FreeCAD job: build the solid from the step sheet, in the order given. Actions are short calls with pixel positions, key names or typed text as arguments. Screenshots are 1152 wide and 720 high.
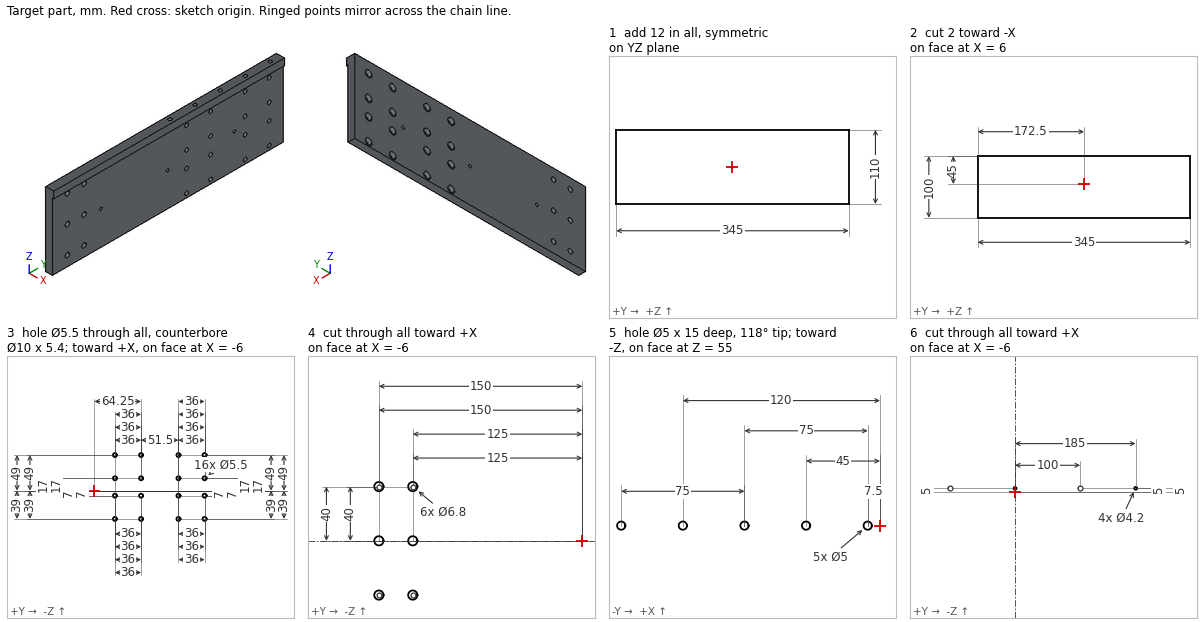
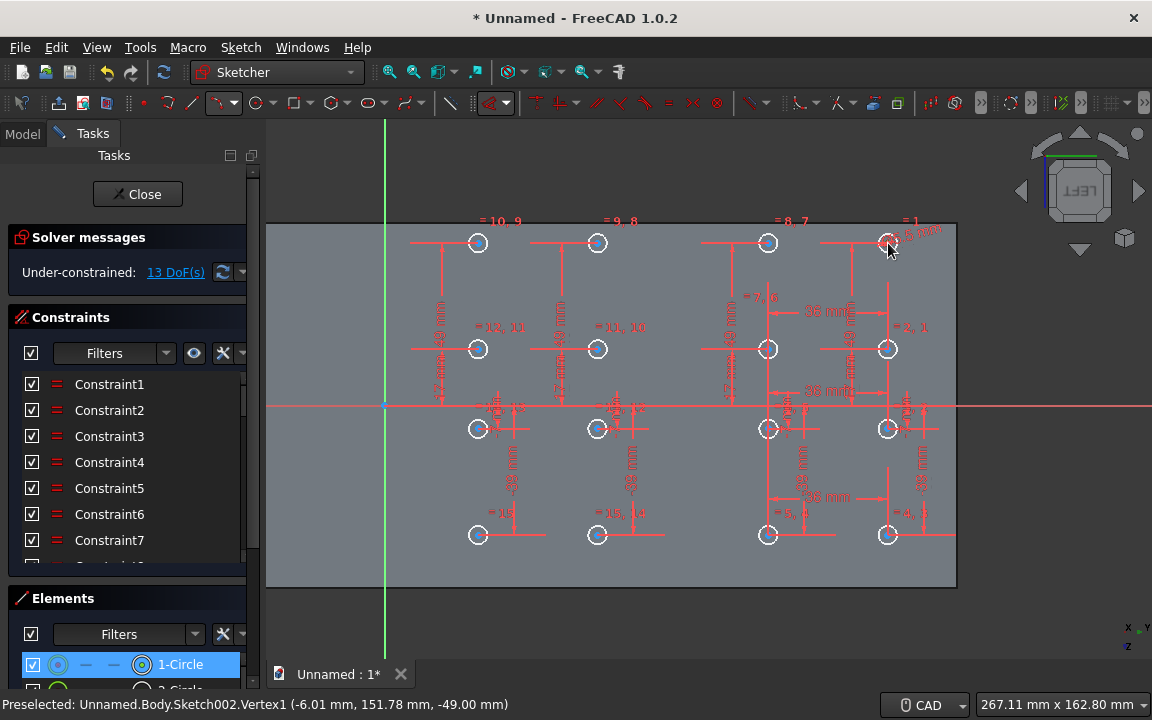
click(768, 535)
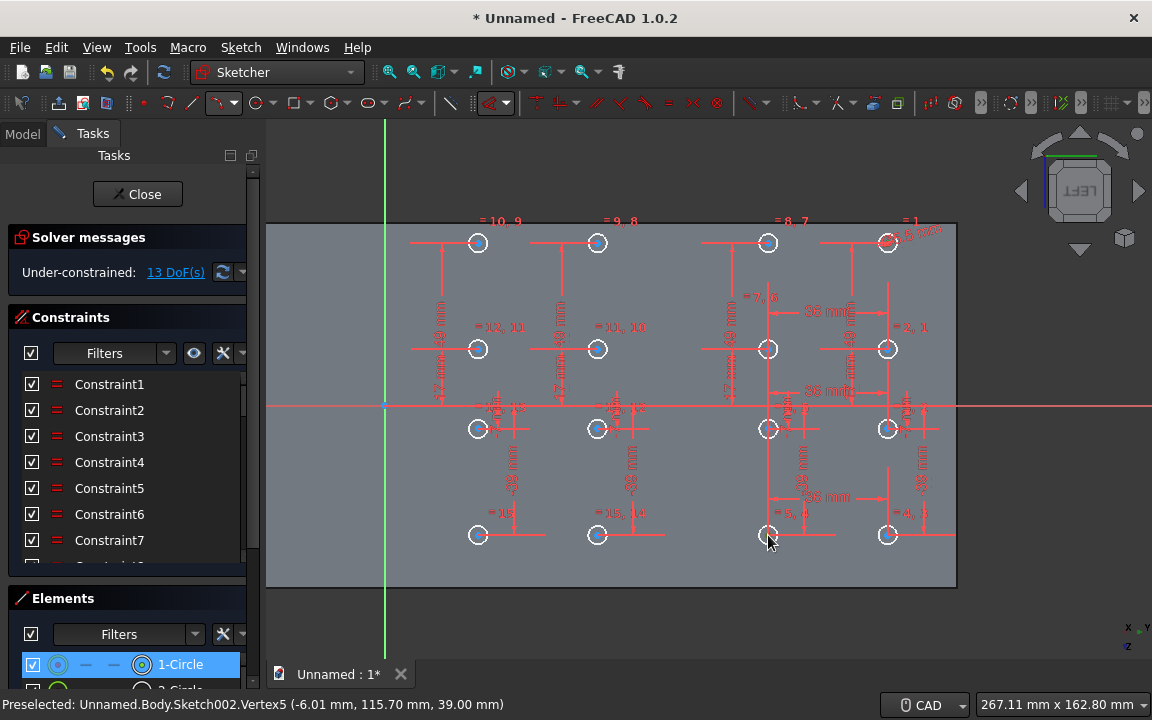
key(l)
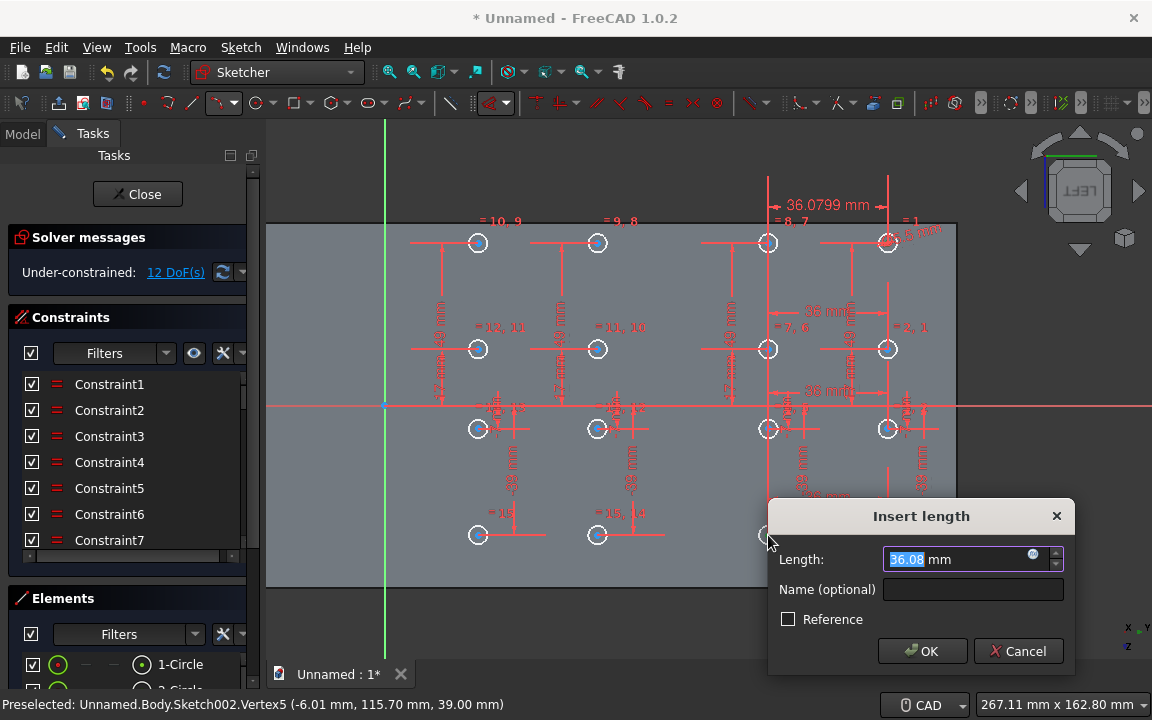
text(36)
key(Return)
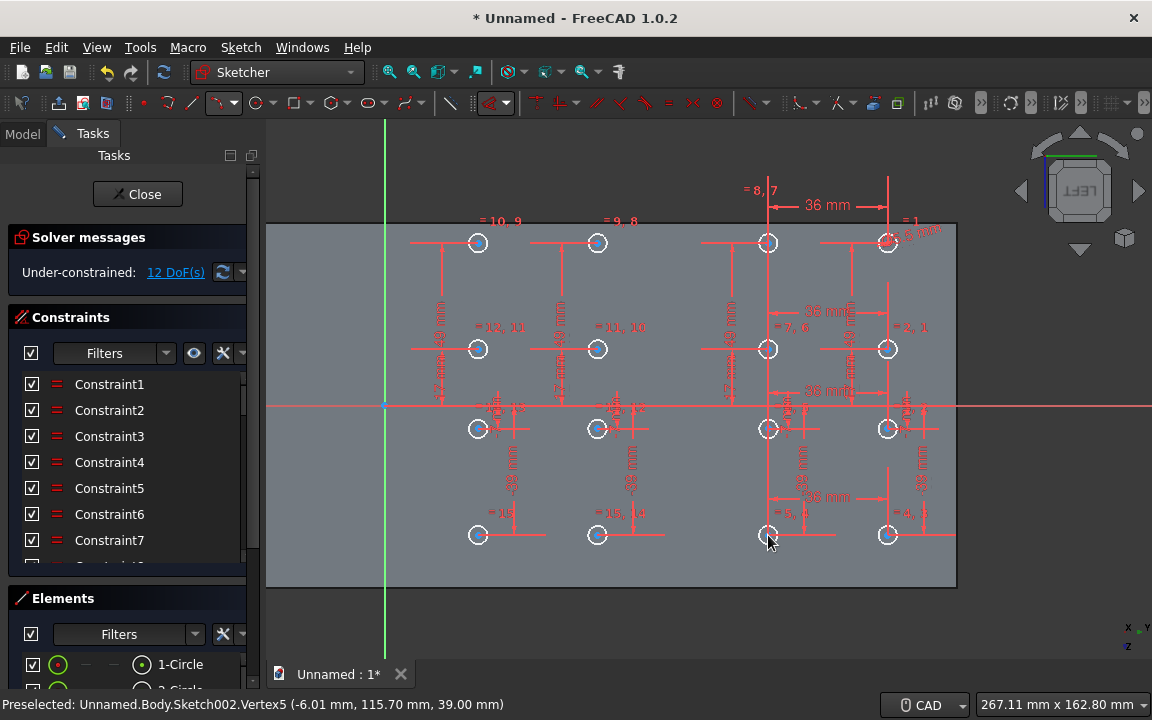
click(888, 429)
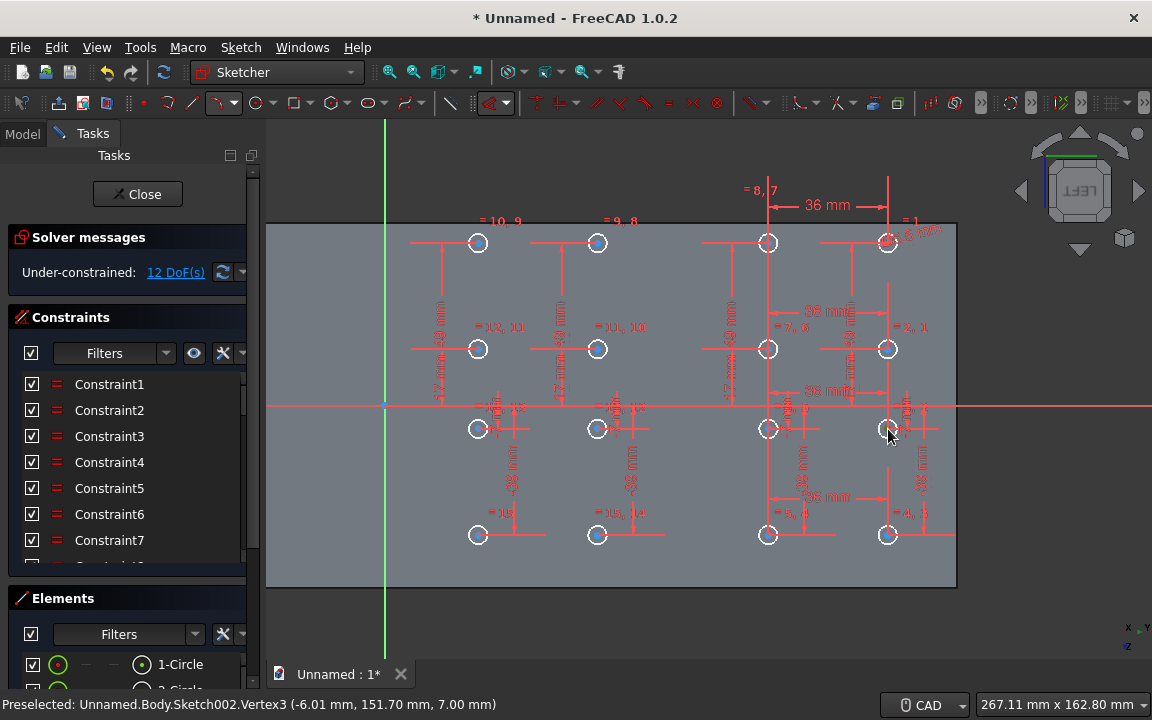
click(769, 429)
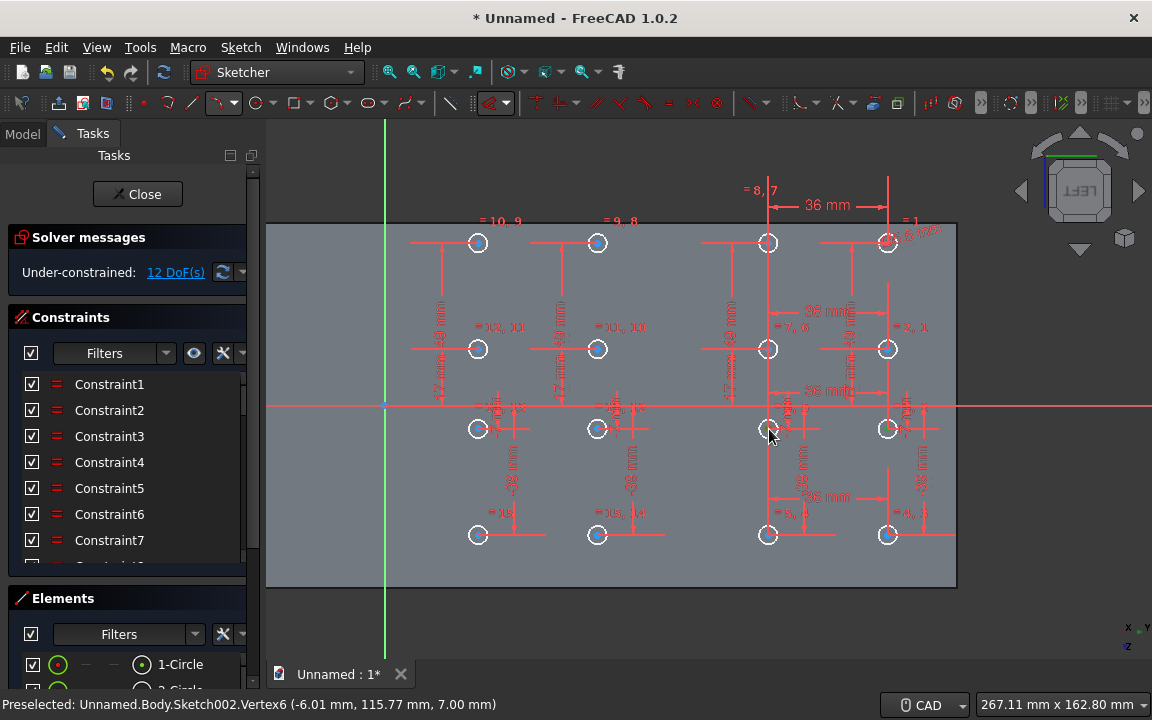
key(l)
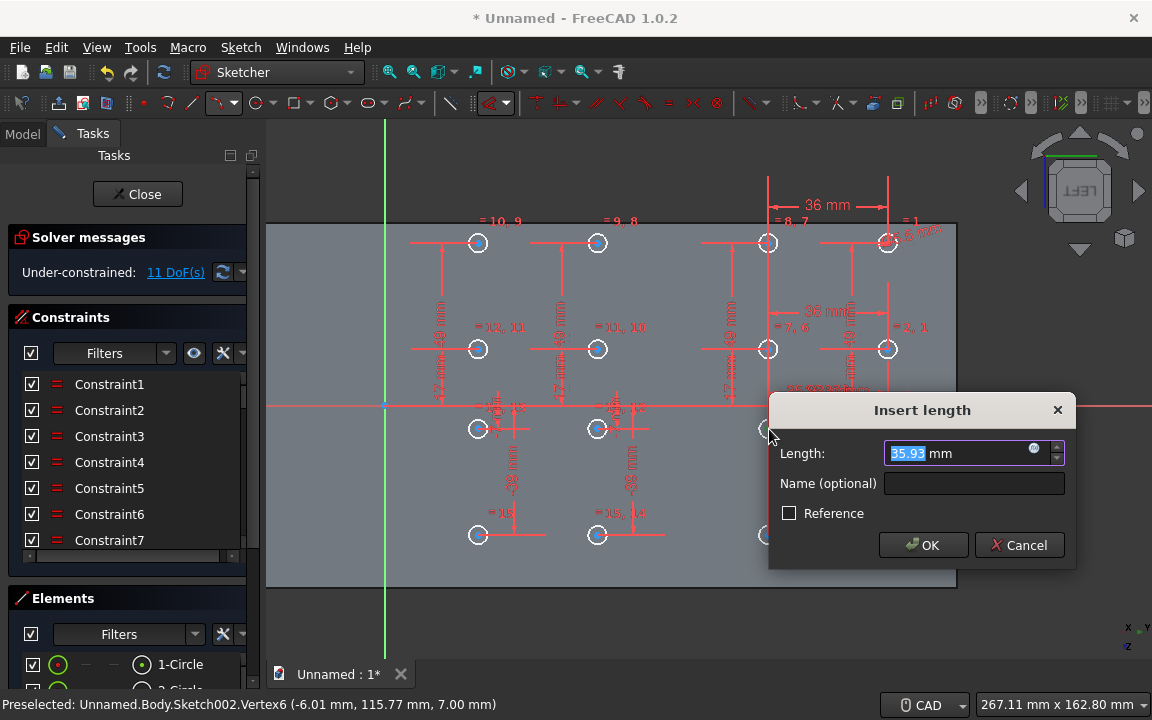
text(36)
key(Return)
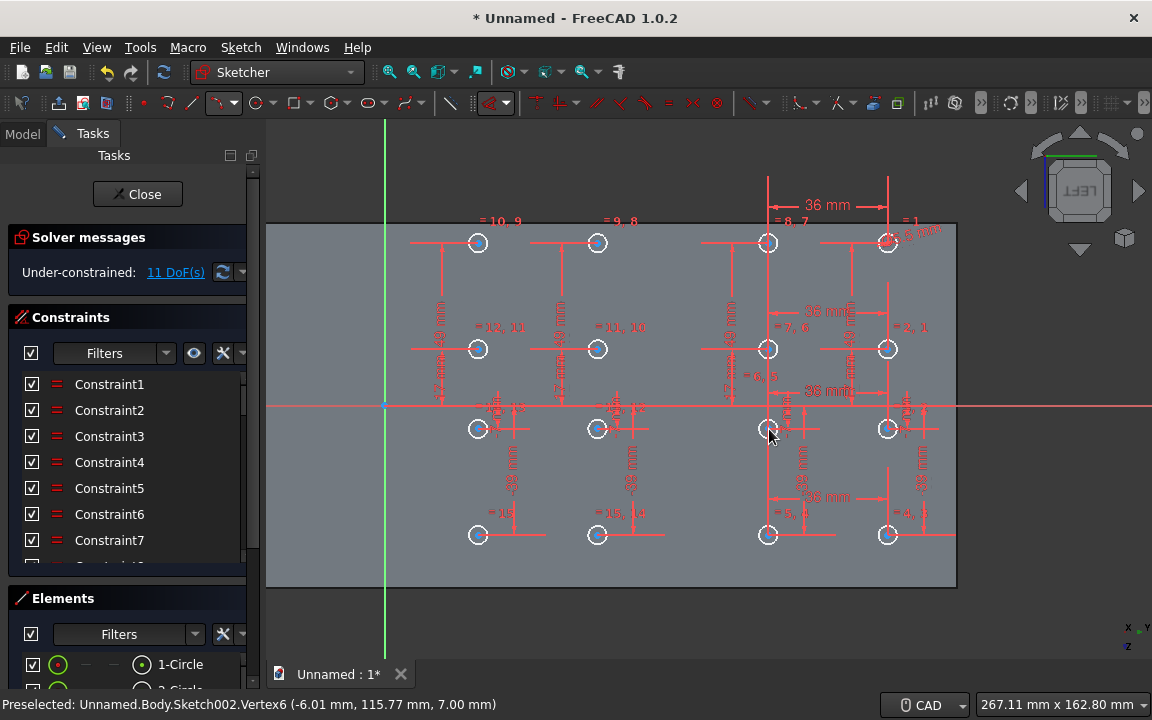
click(888, 349)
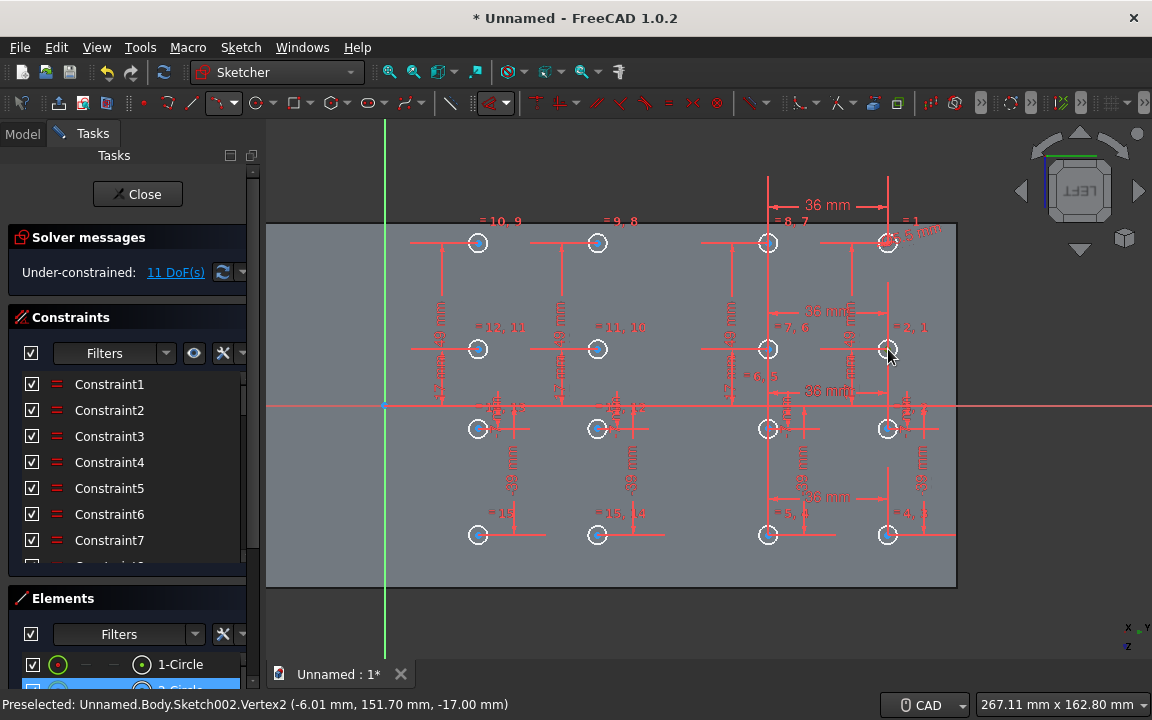
click(768, 349)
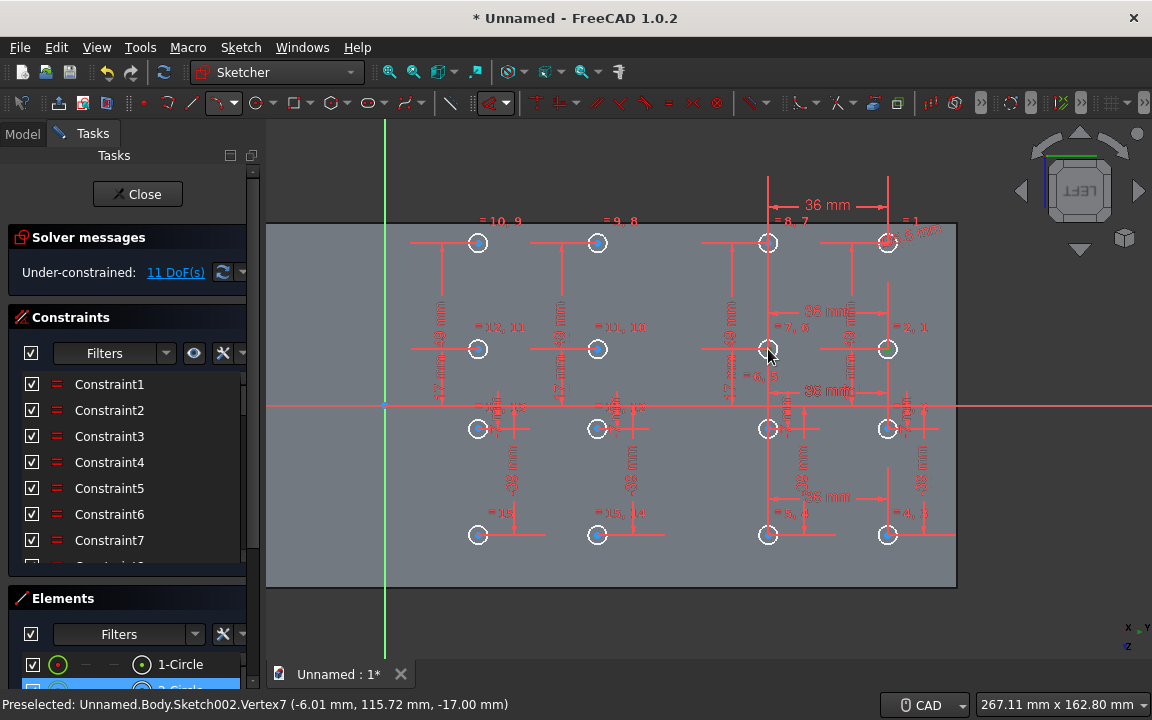
key(l)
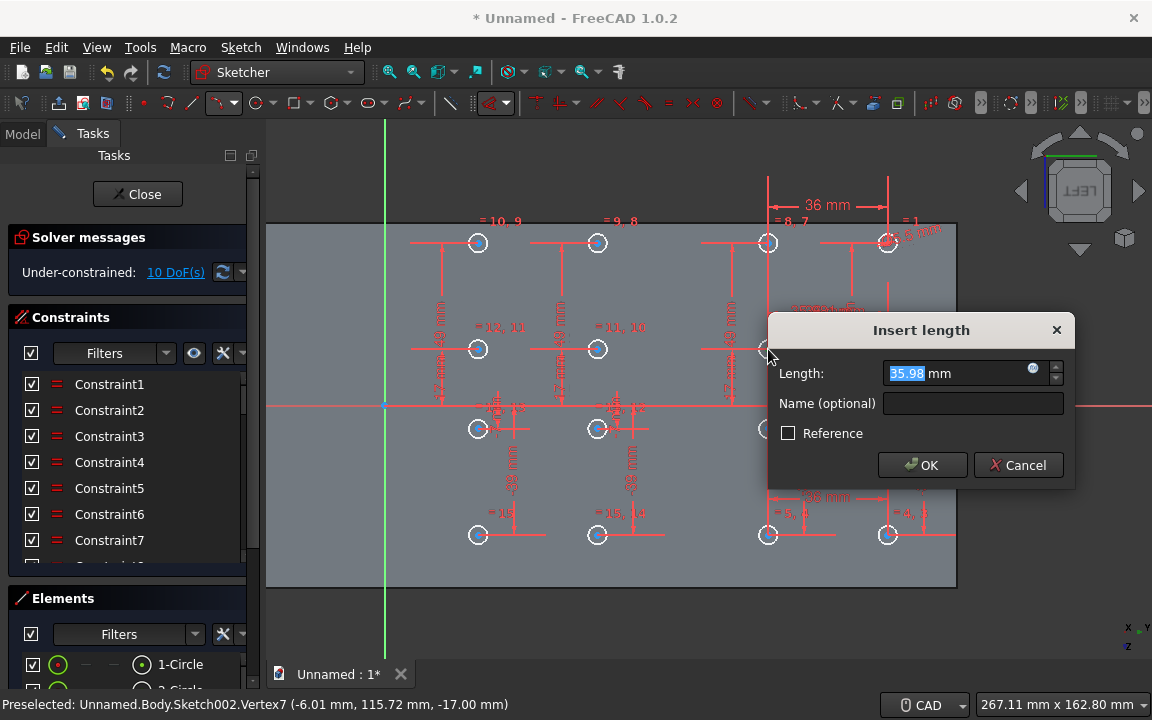
text(36)
key(Return)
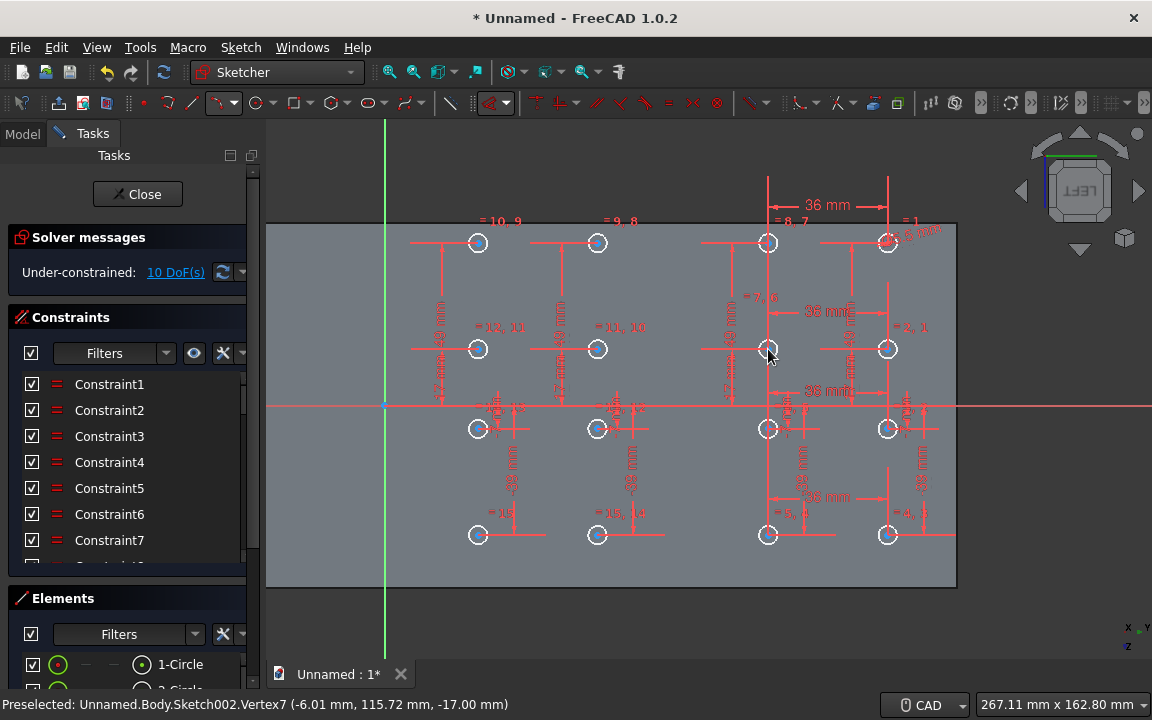
click(888, 243)